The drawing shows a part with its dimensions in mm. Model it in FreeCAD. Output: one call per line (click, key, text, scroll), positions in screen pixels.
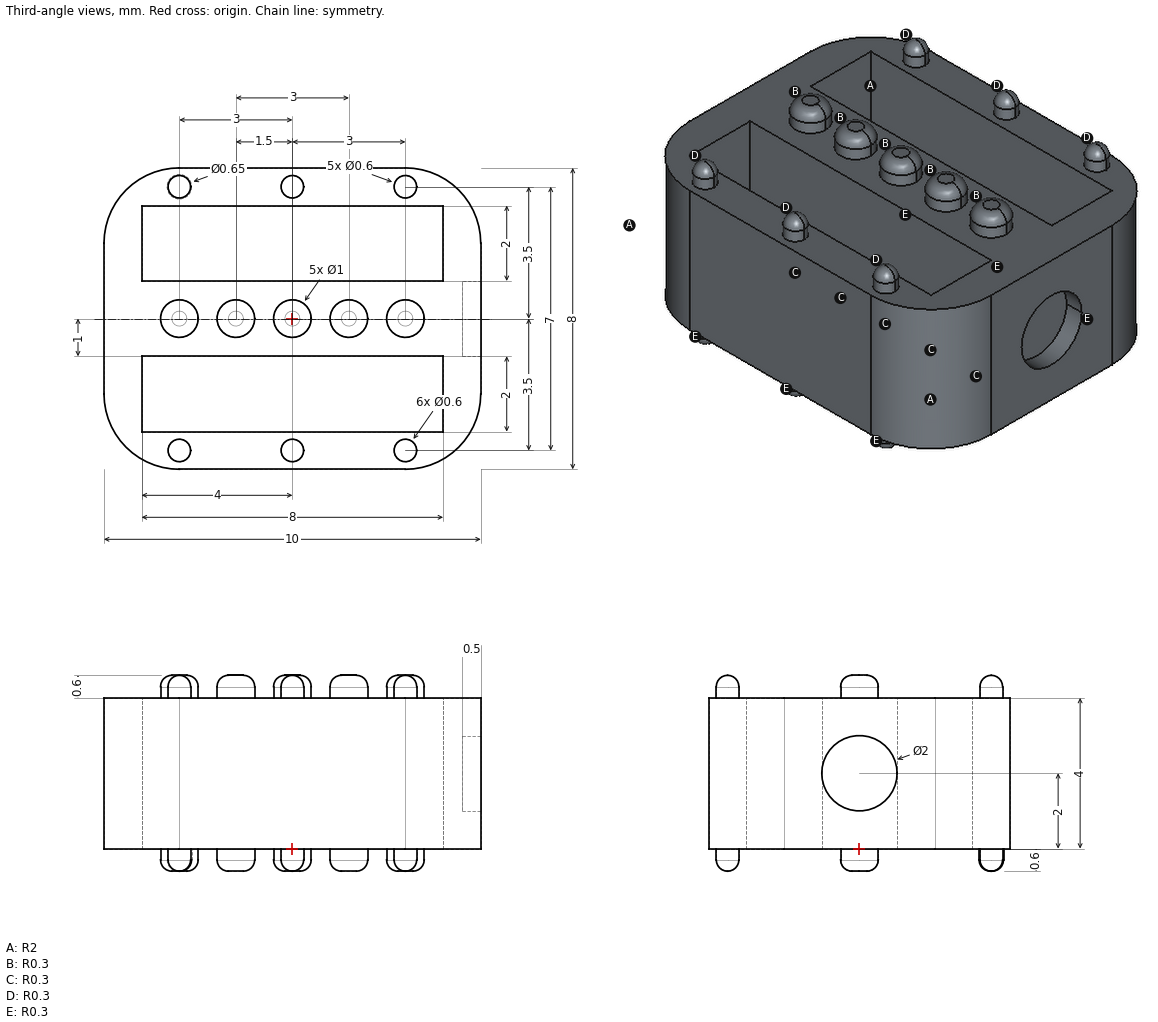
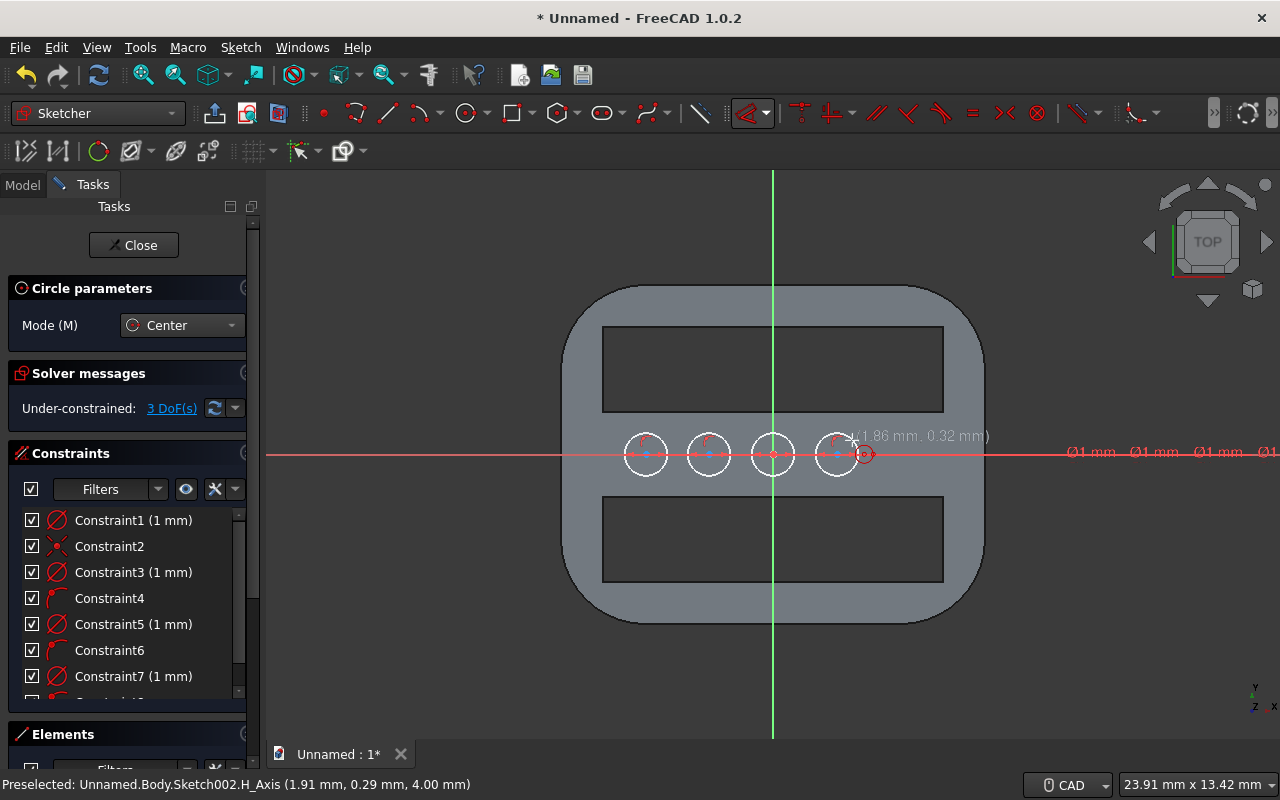
click(900, 455)
move(915, 440)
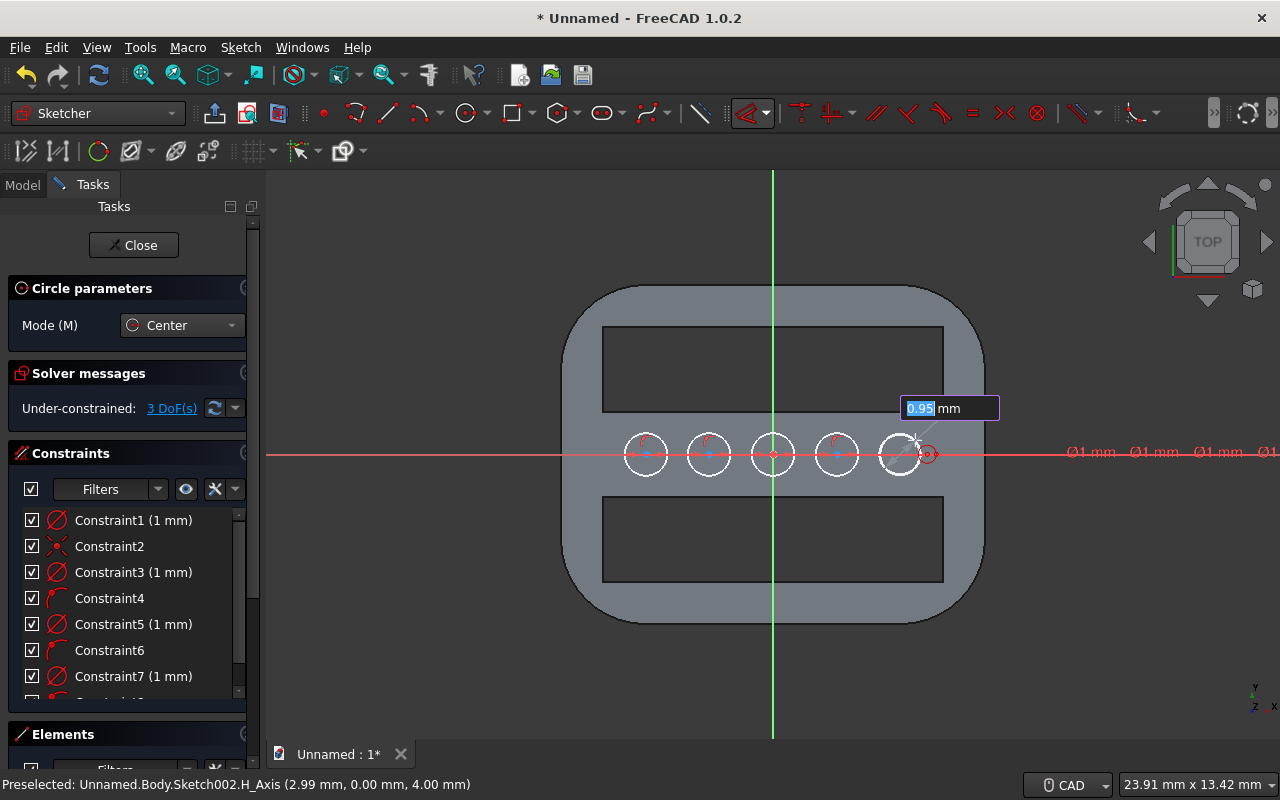
text(1)
key(Return)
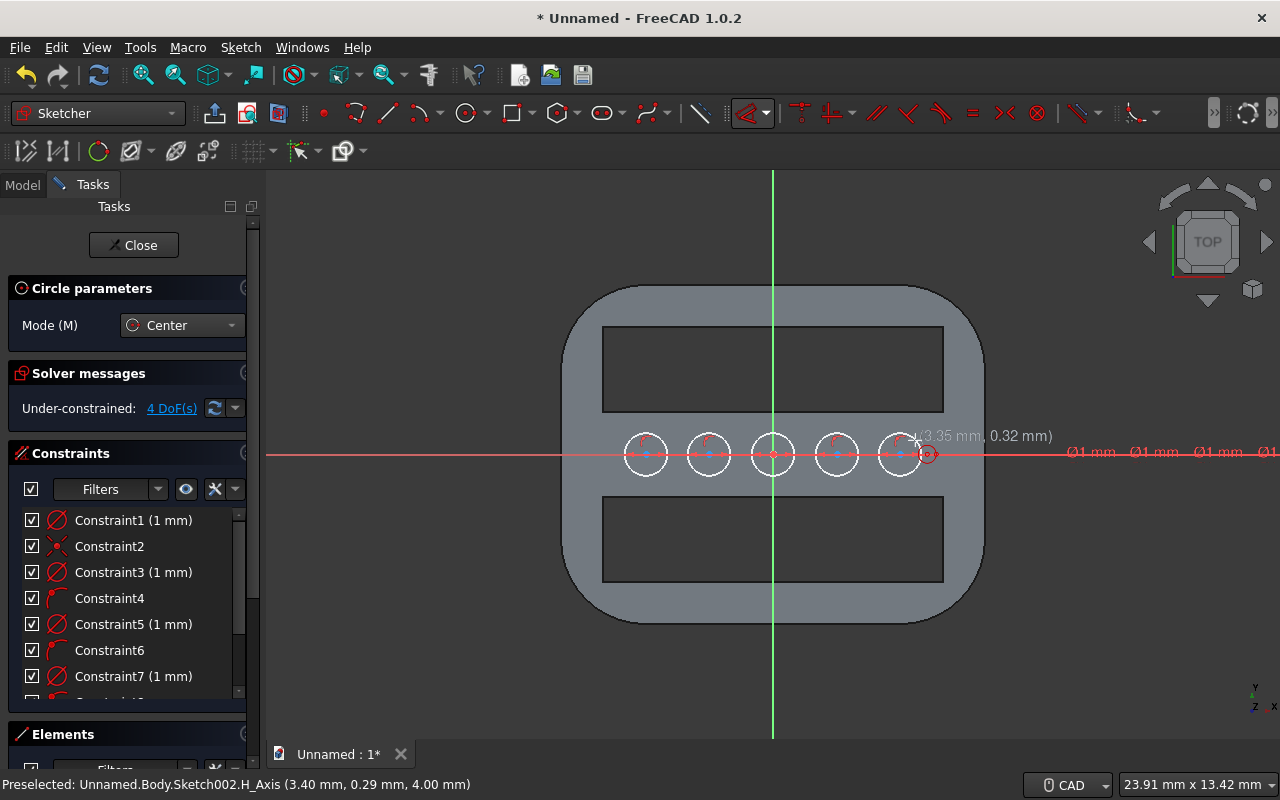
scroll(900, 603, up, 3)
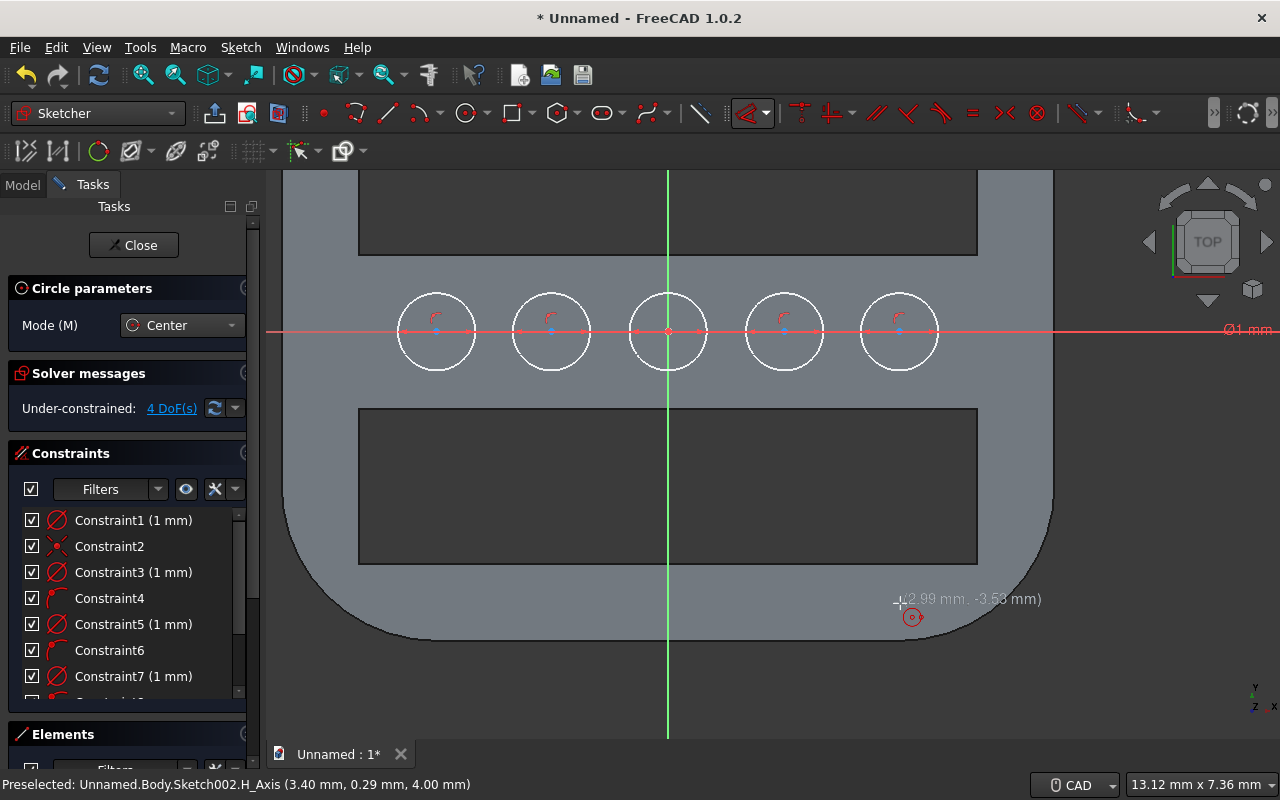
click(900, 602)
move(916, 586)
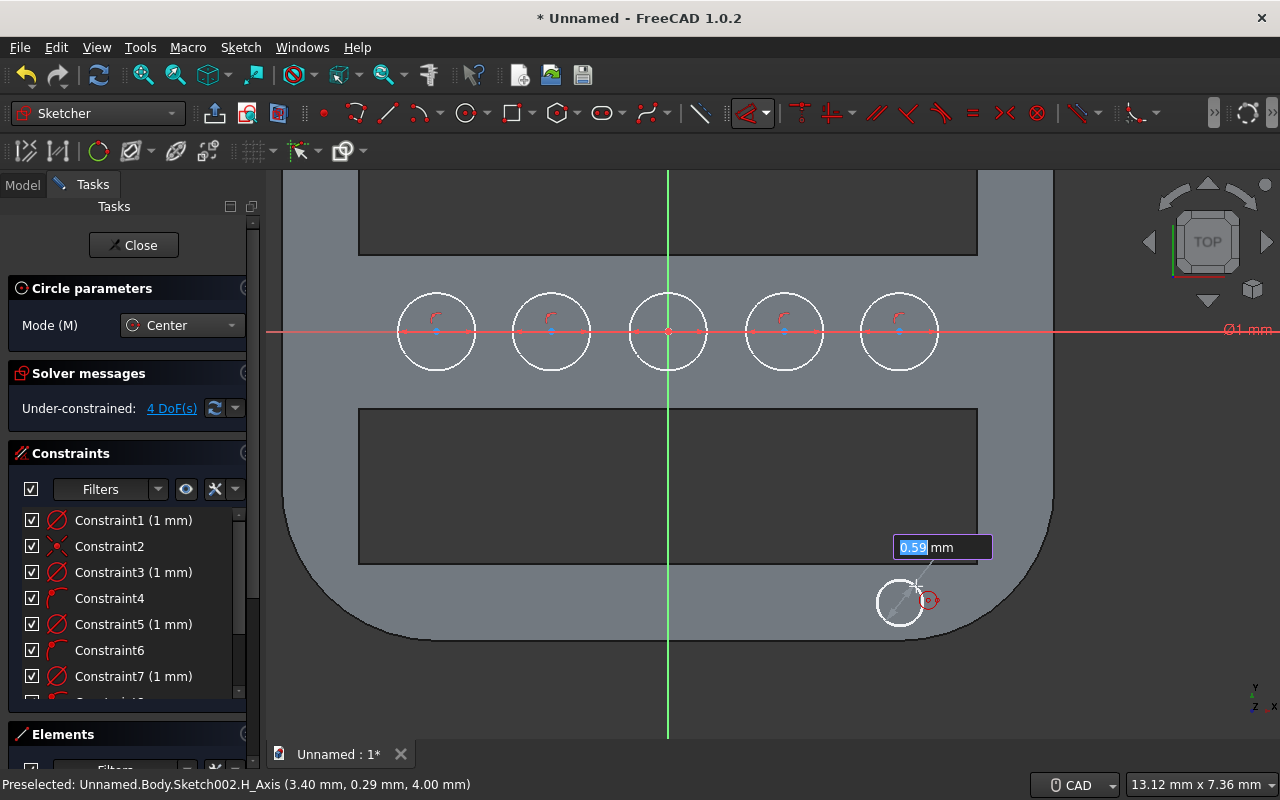
text(0.6)
key(Return)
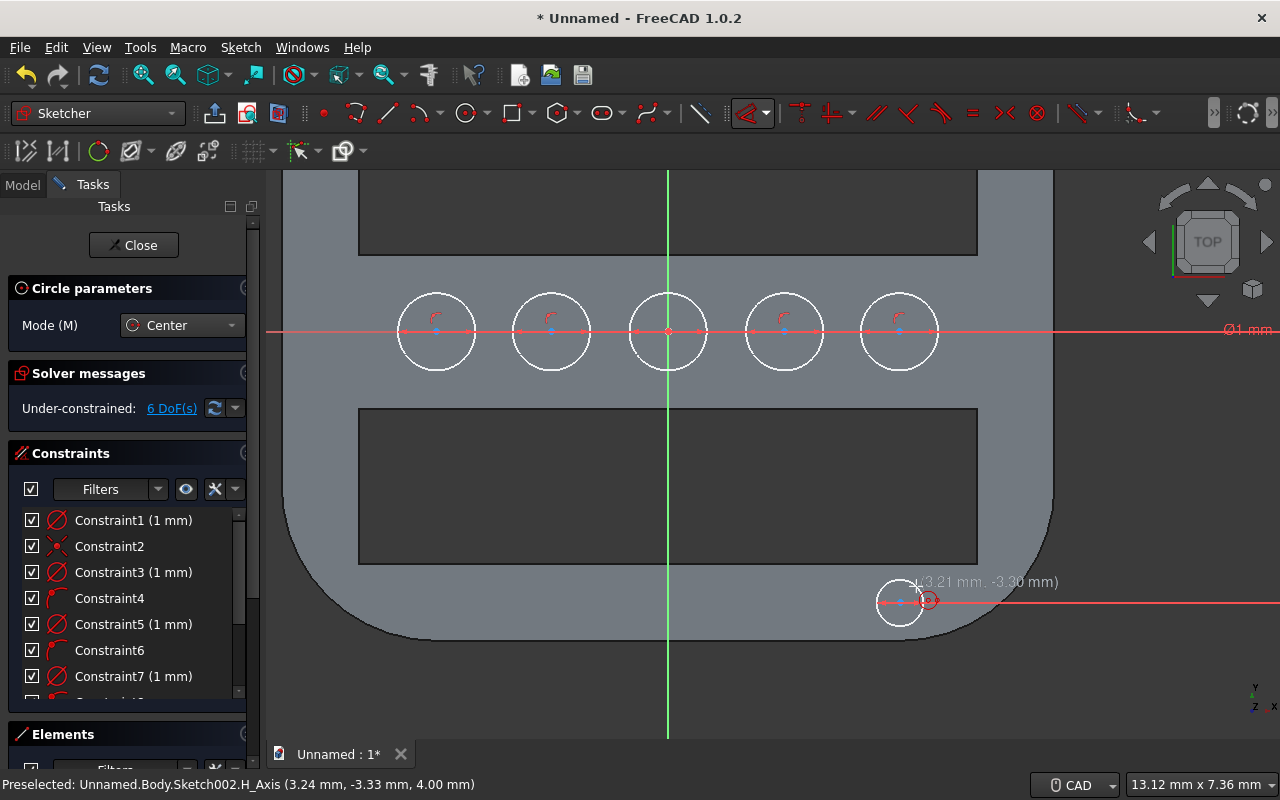
click(668, 602)
move(684, 586)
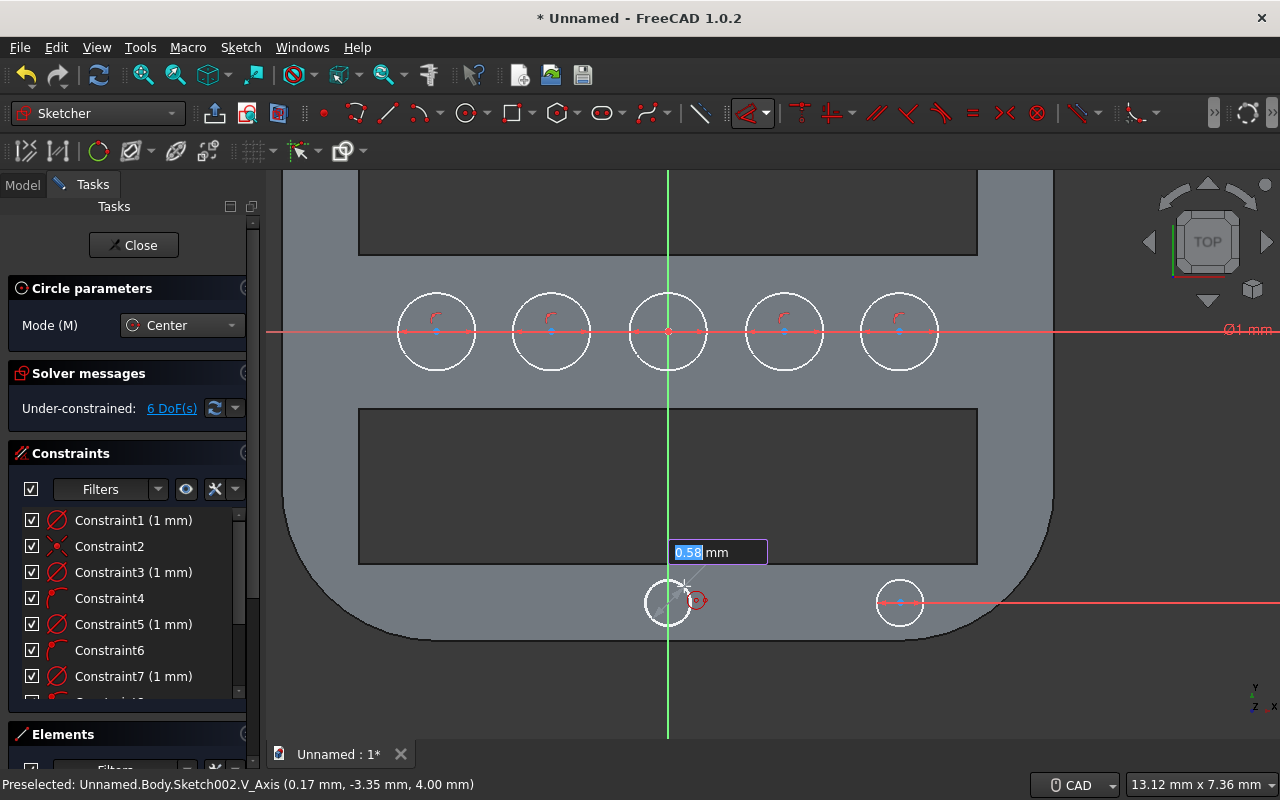
text(0.6)
key(Return)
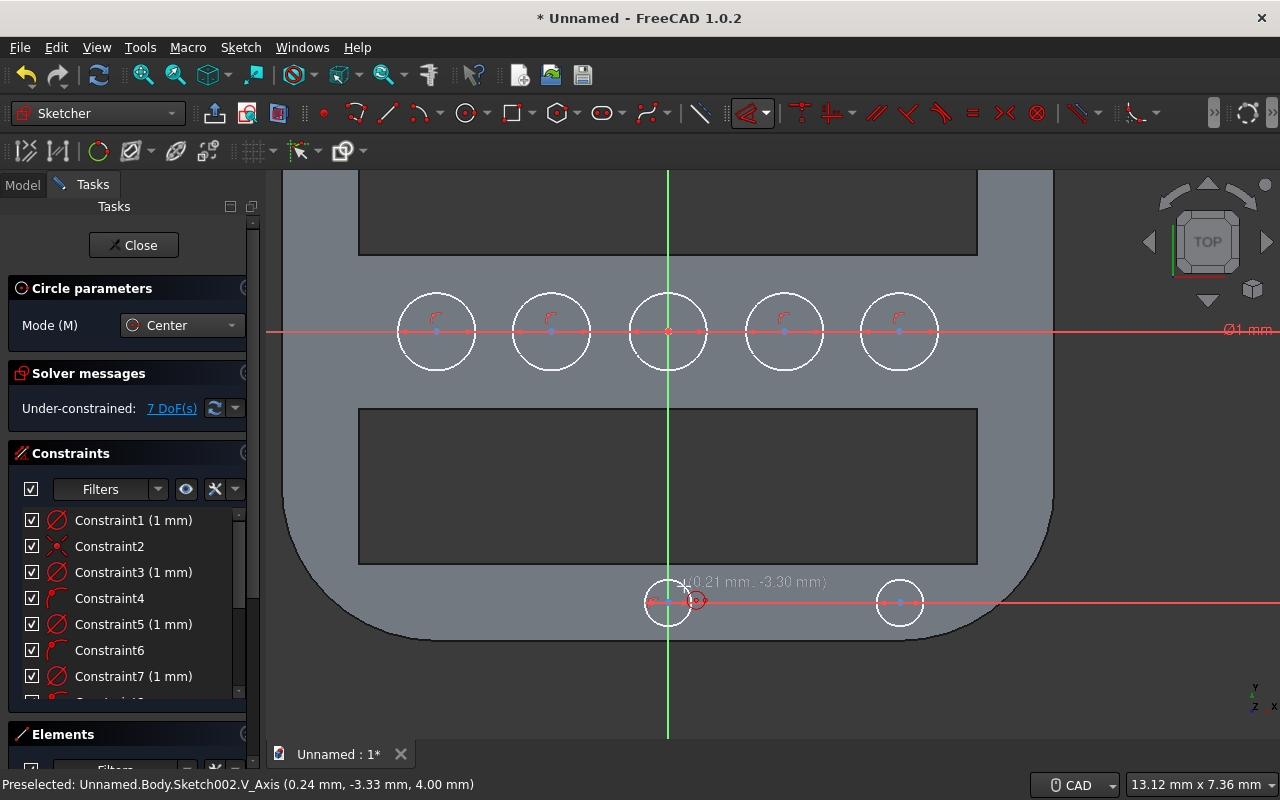
click(436, 602)
move(453, 586)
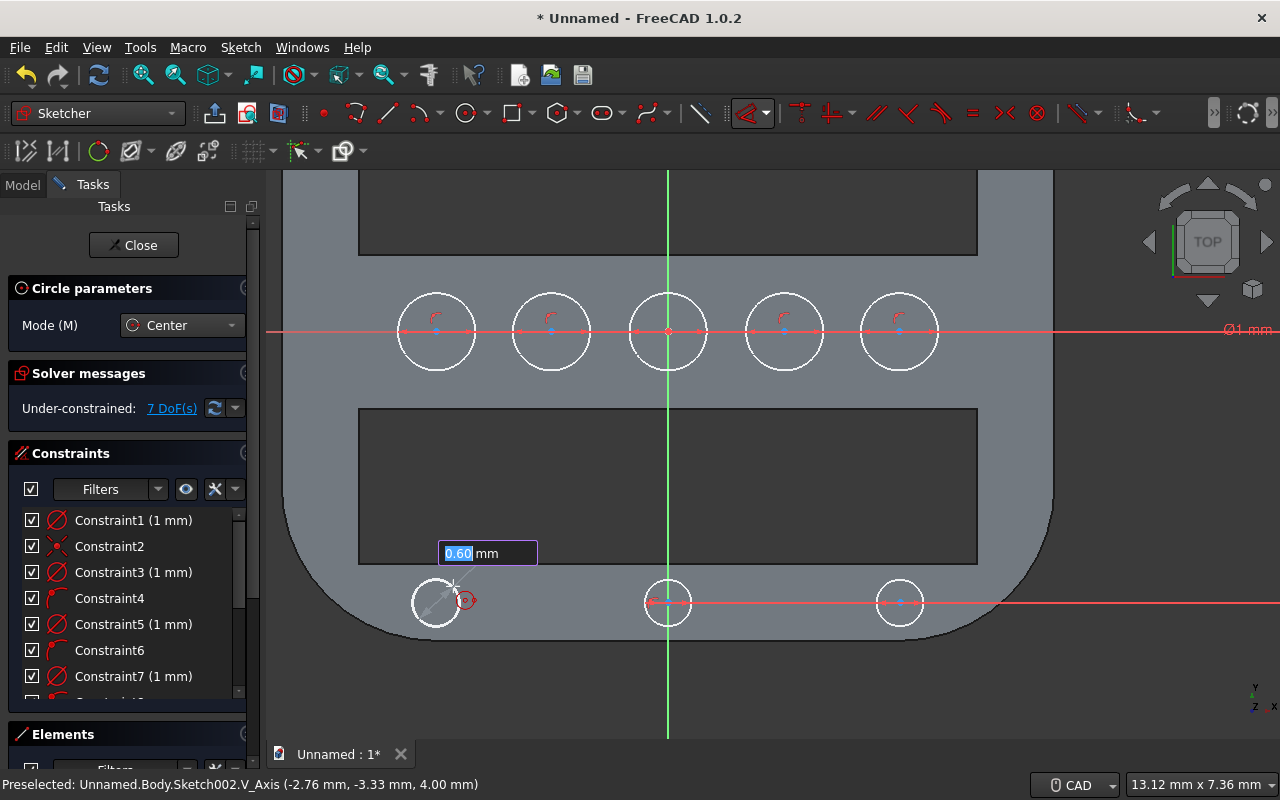
text(0.6)
key(Return)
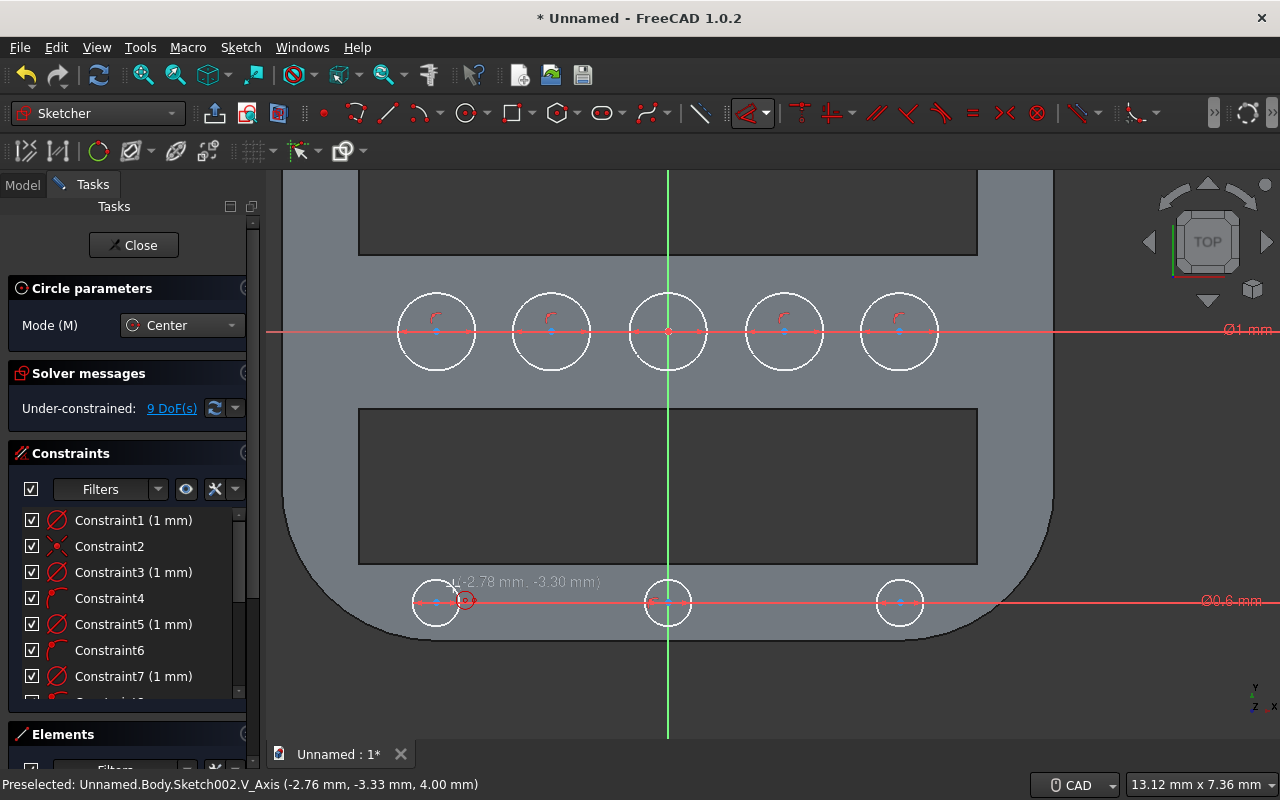
scroll(779, 704, down, 2)